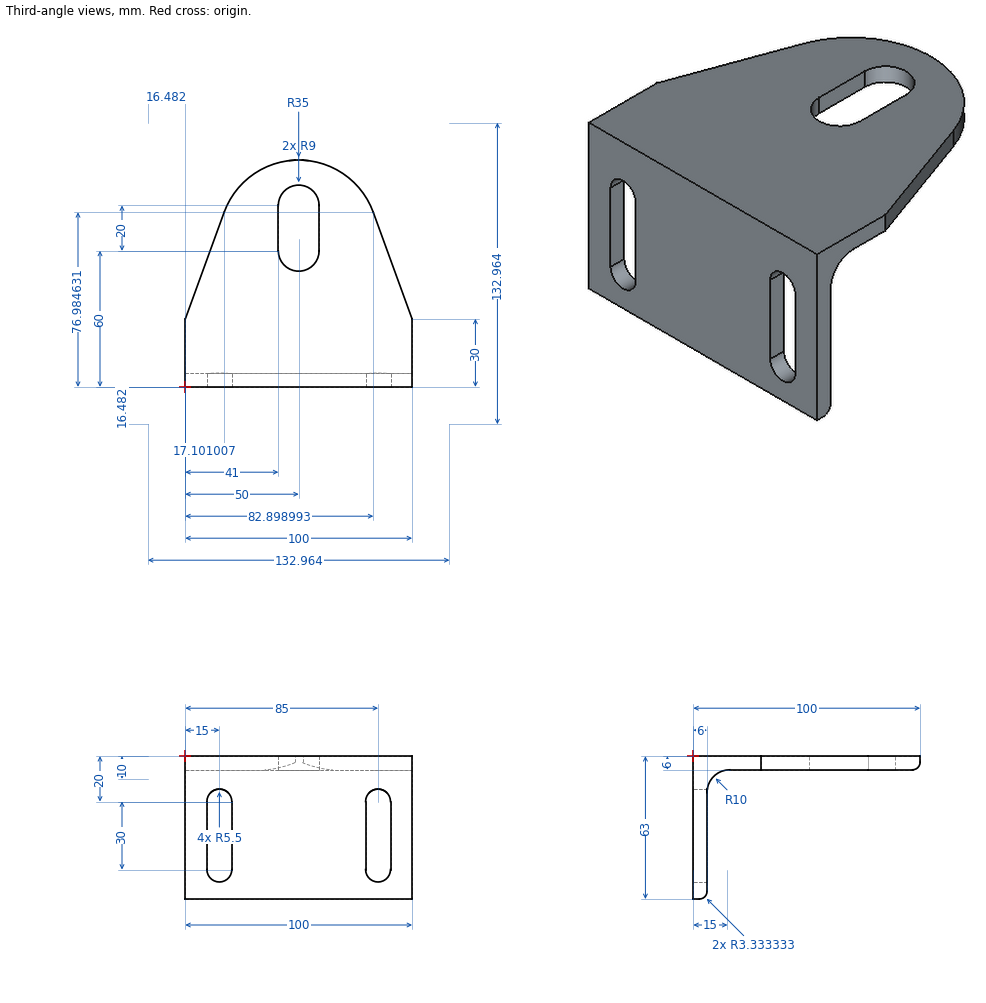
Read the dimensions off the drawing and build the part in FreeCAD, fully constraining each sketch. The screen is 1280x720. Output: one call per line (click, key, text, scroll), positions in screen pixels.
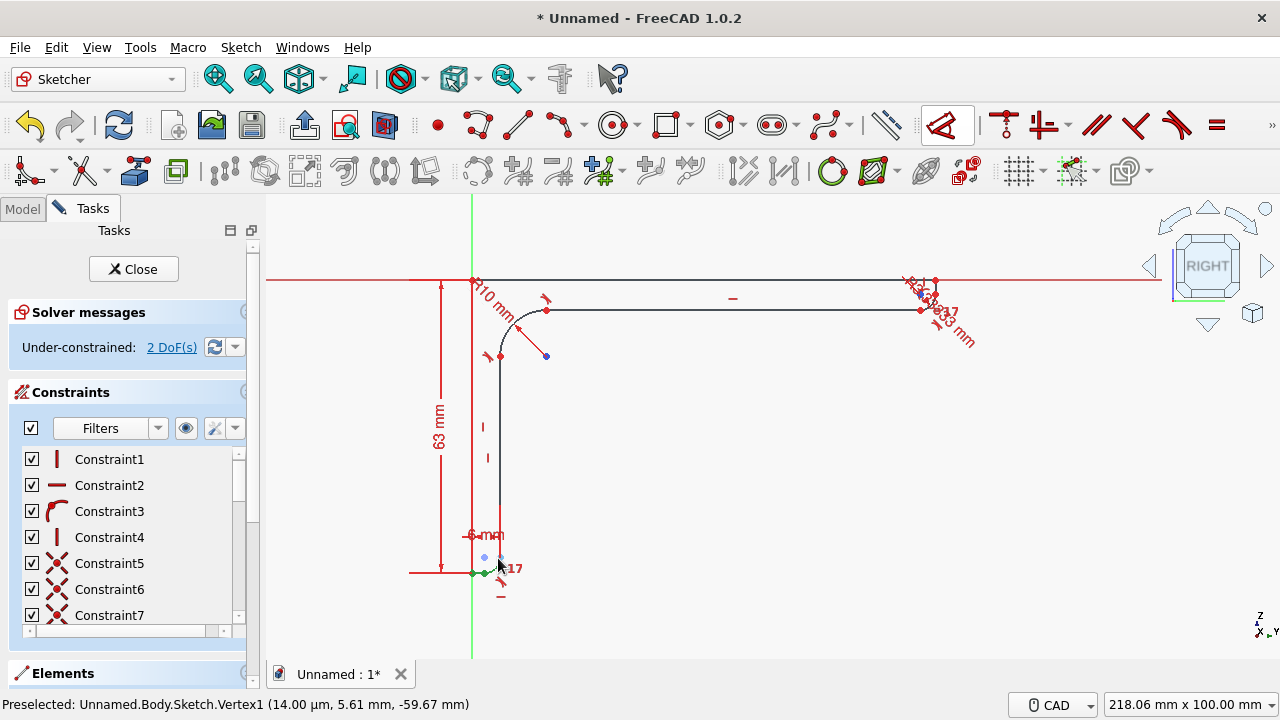
scroll(547, 310, up, 2)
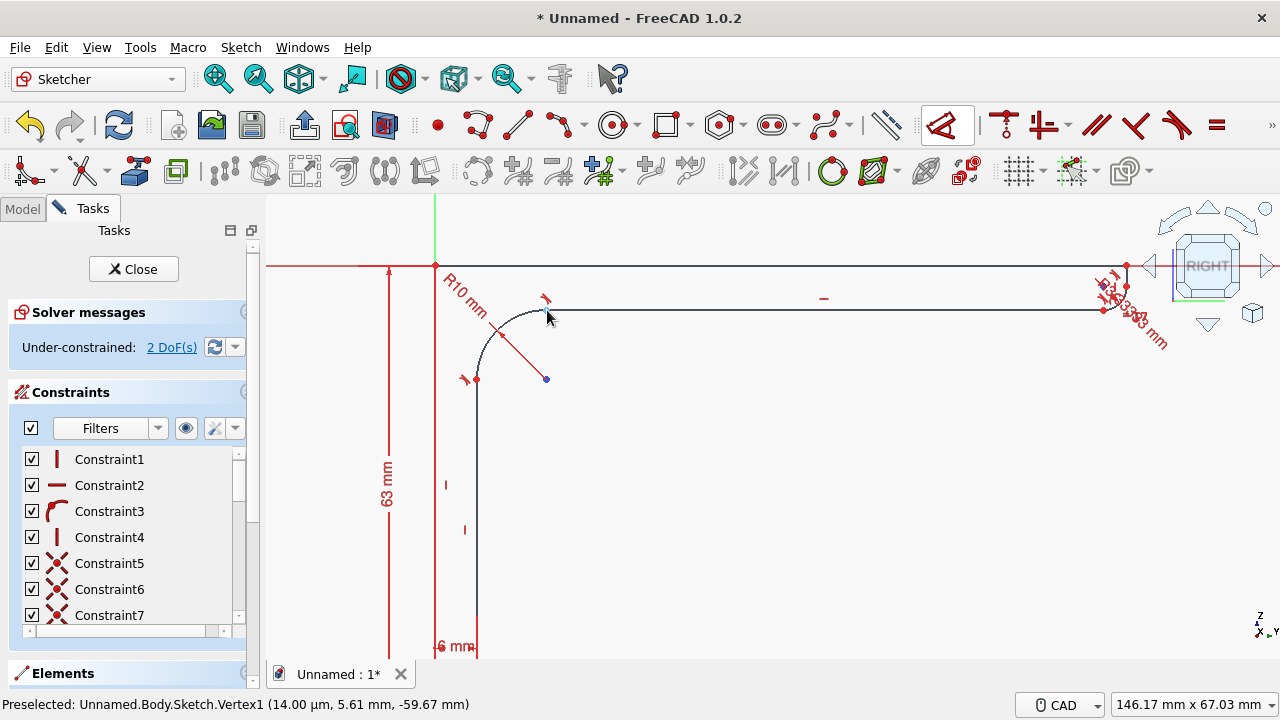
click(546, 310)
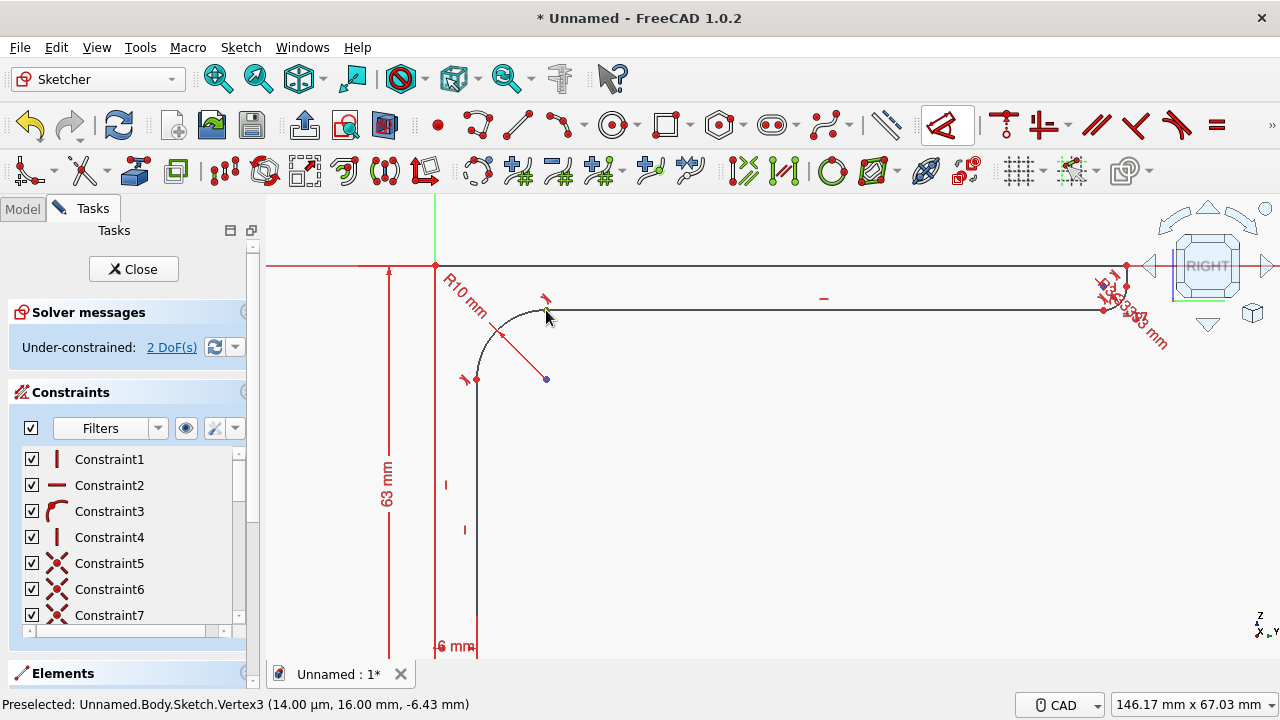
click(968, 126)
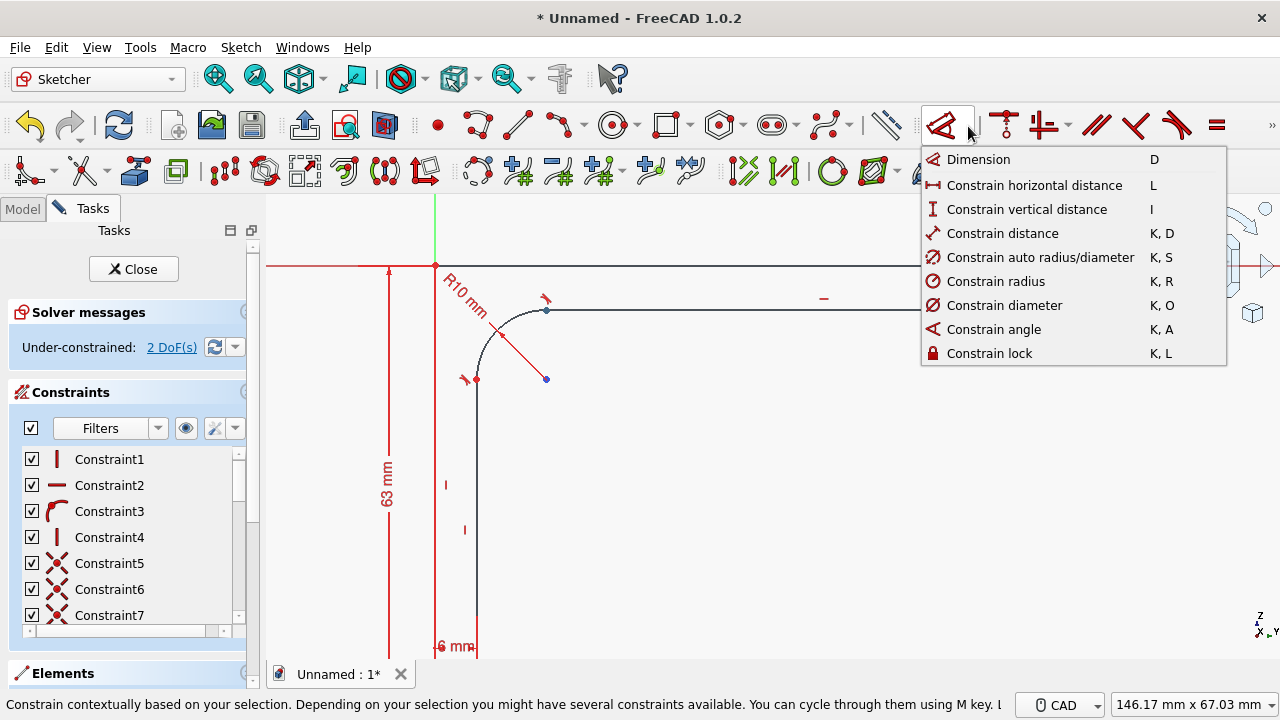
click(1074, 209)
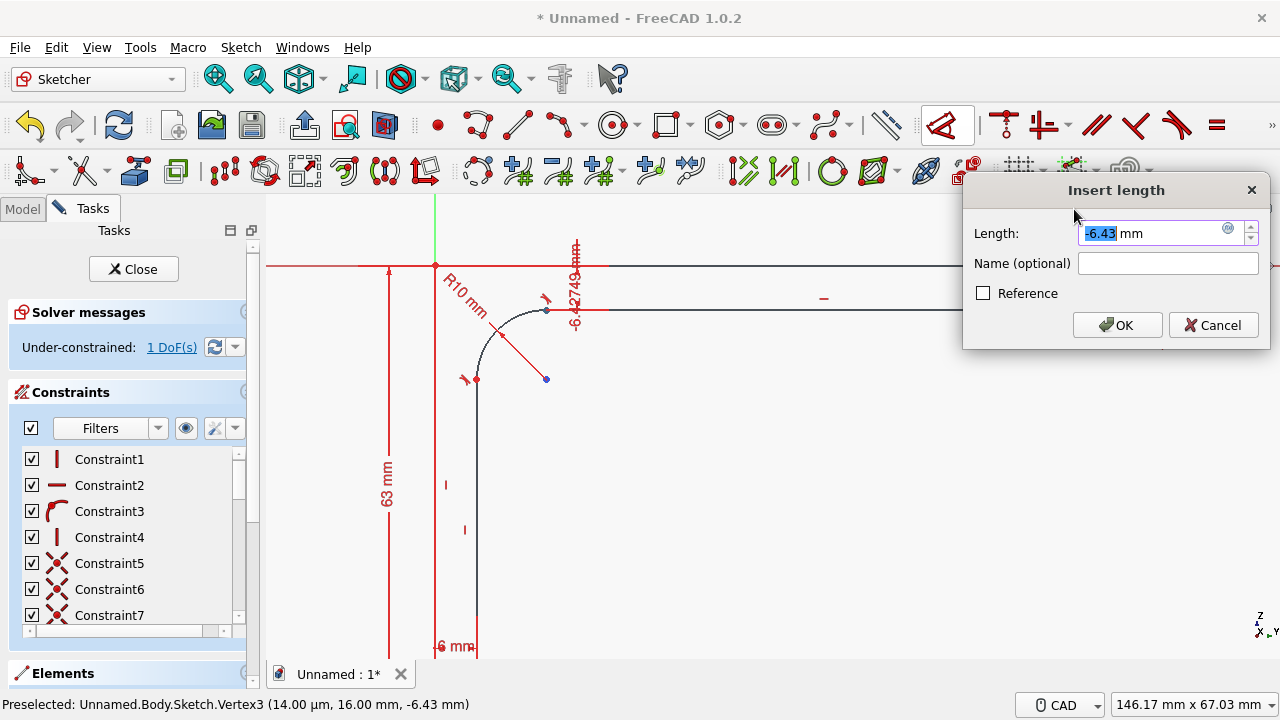
text(-6)
key(Return)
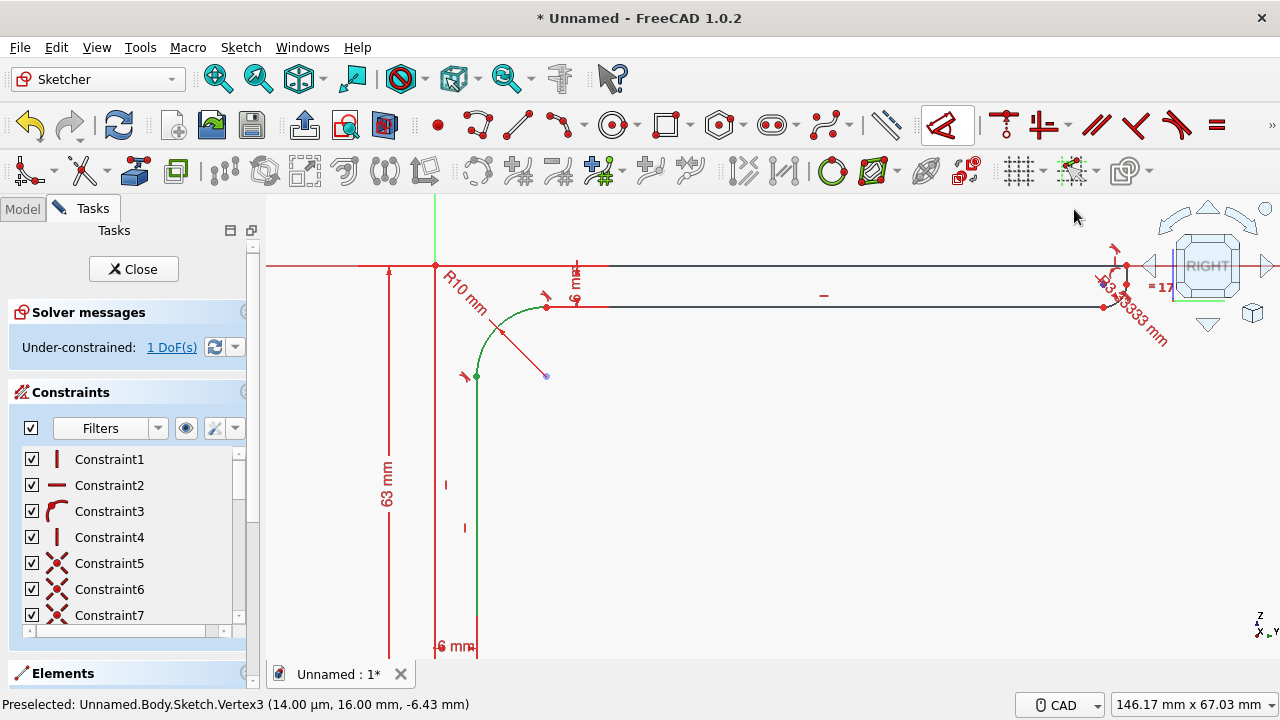
click(919, 266)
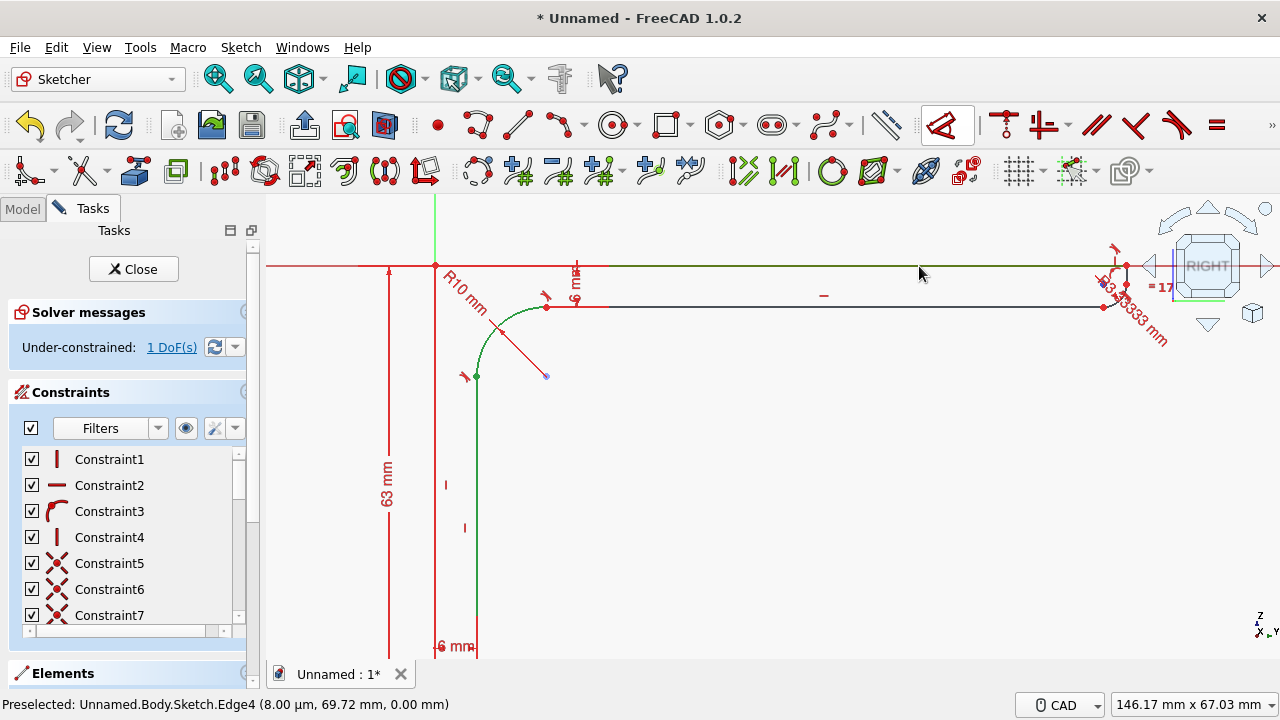
click(968, 126)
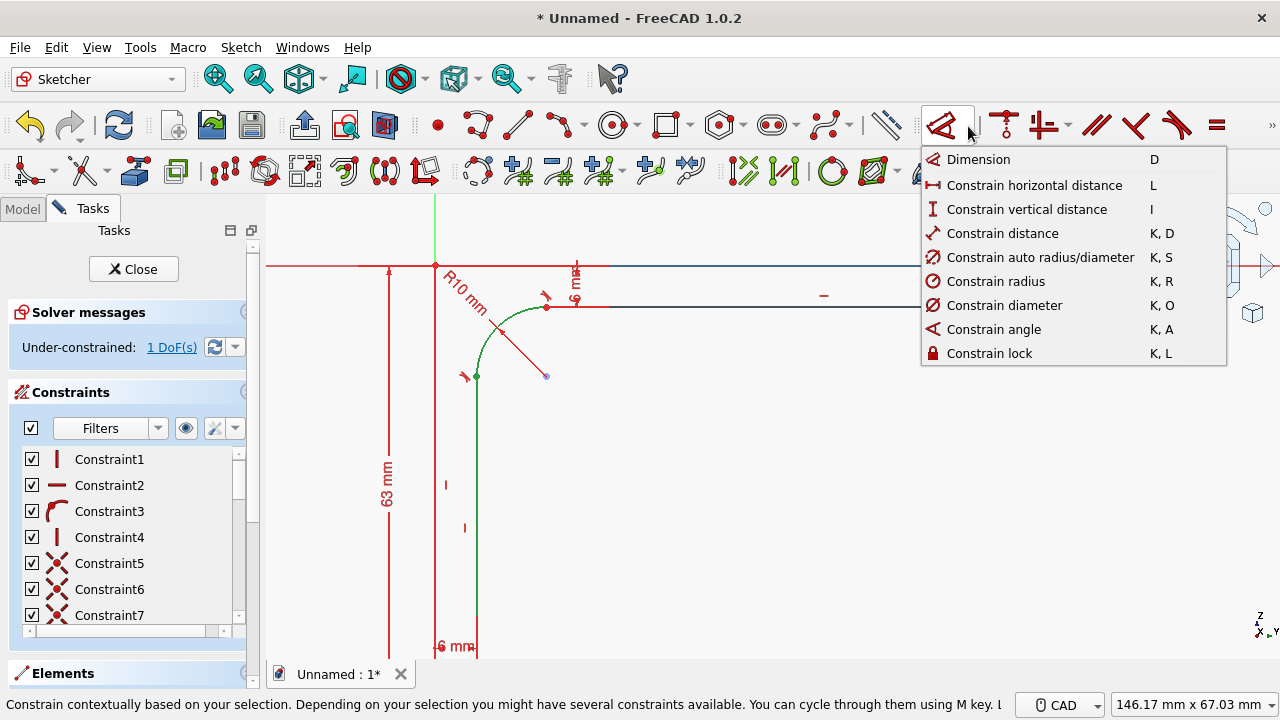
click(1074, 185)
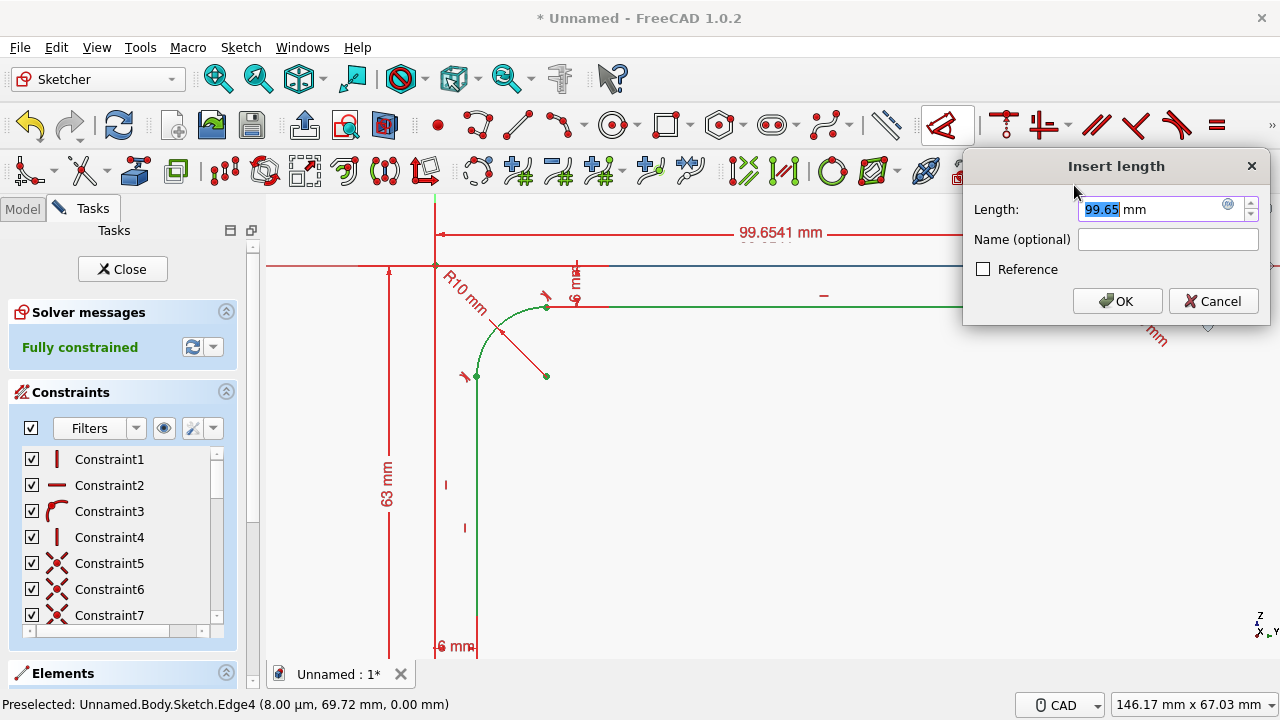
text(100)
key(Return)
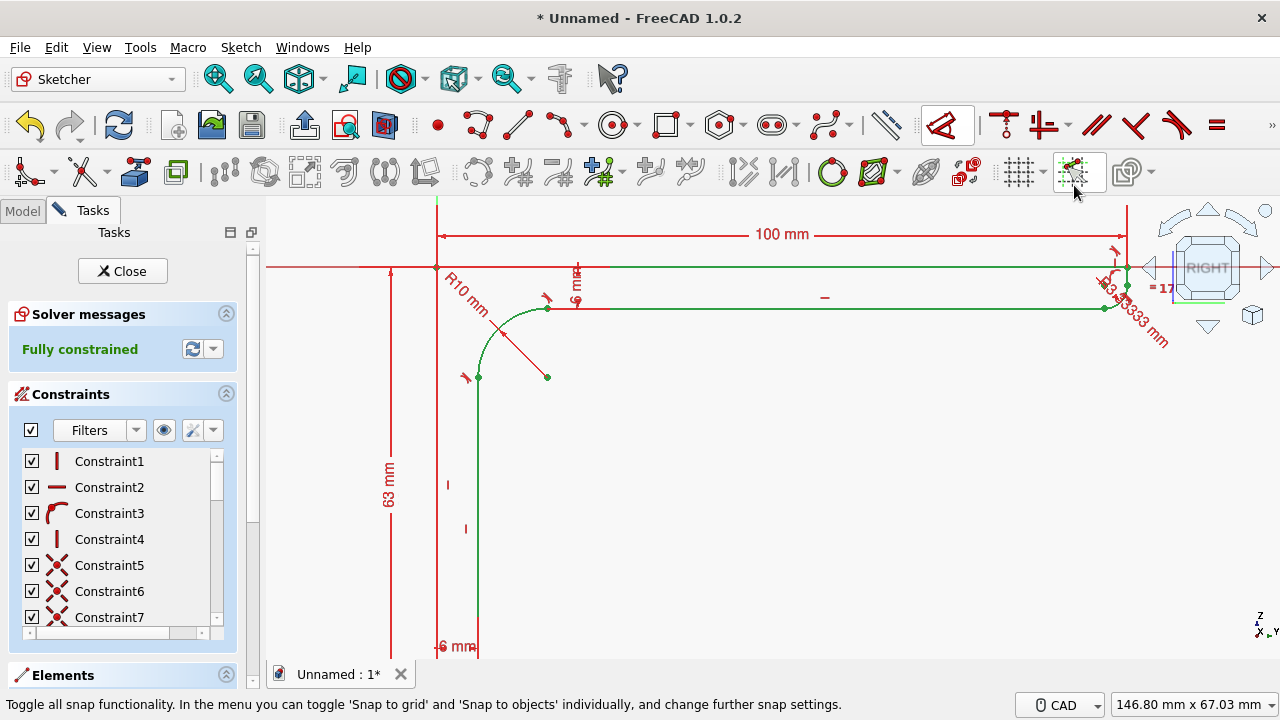
click(123, 271)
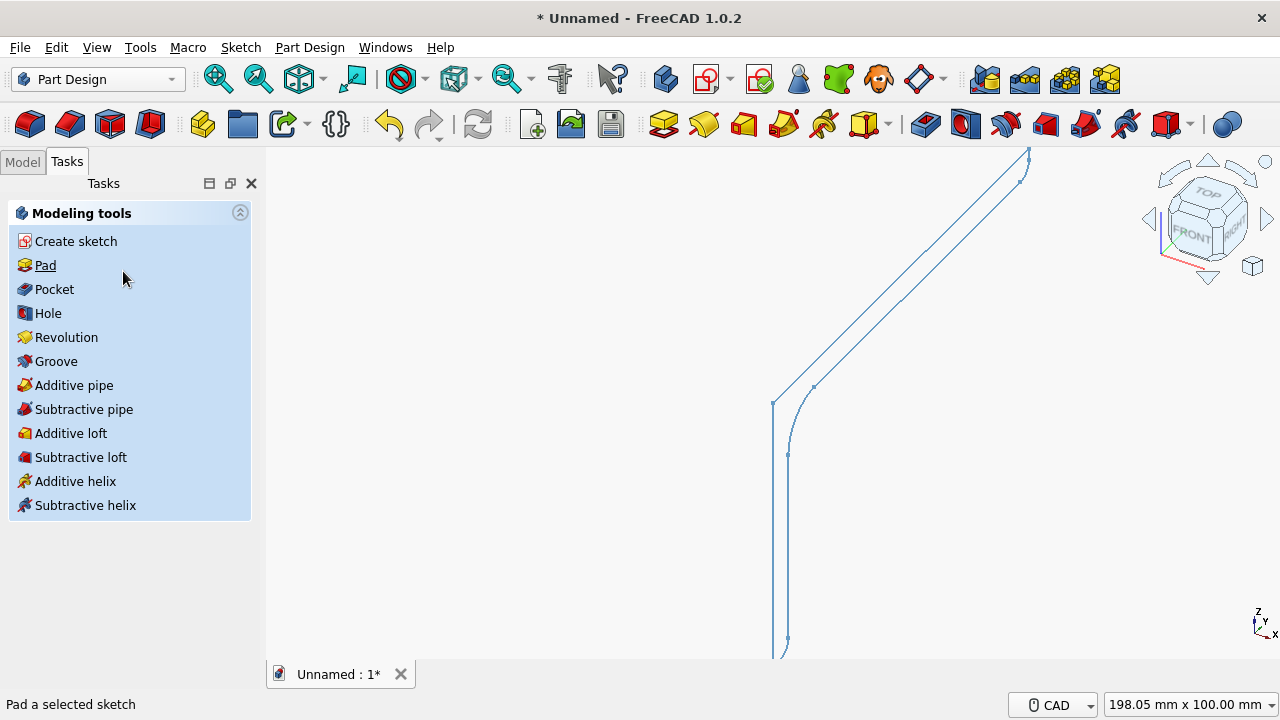
click(664, 124)